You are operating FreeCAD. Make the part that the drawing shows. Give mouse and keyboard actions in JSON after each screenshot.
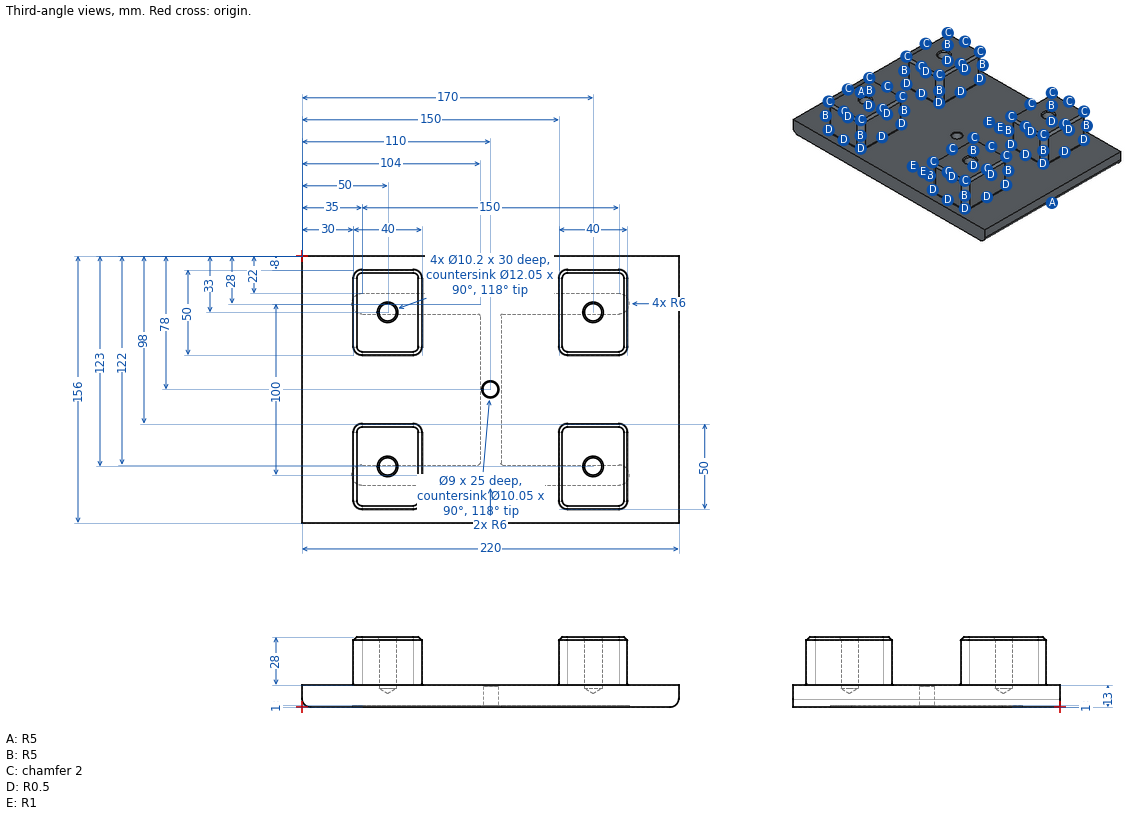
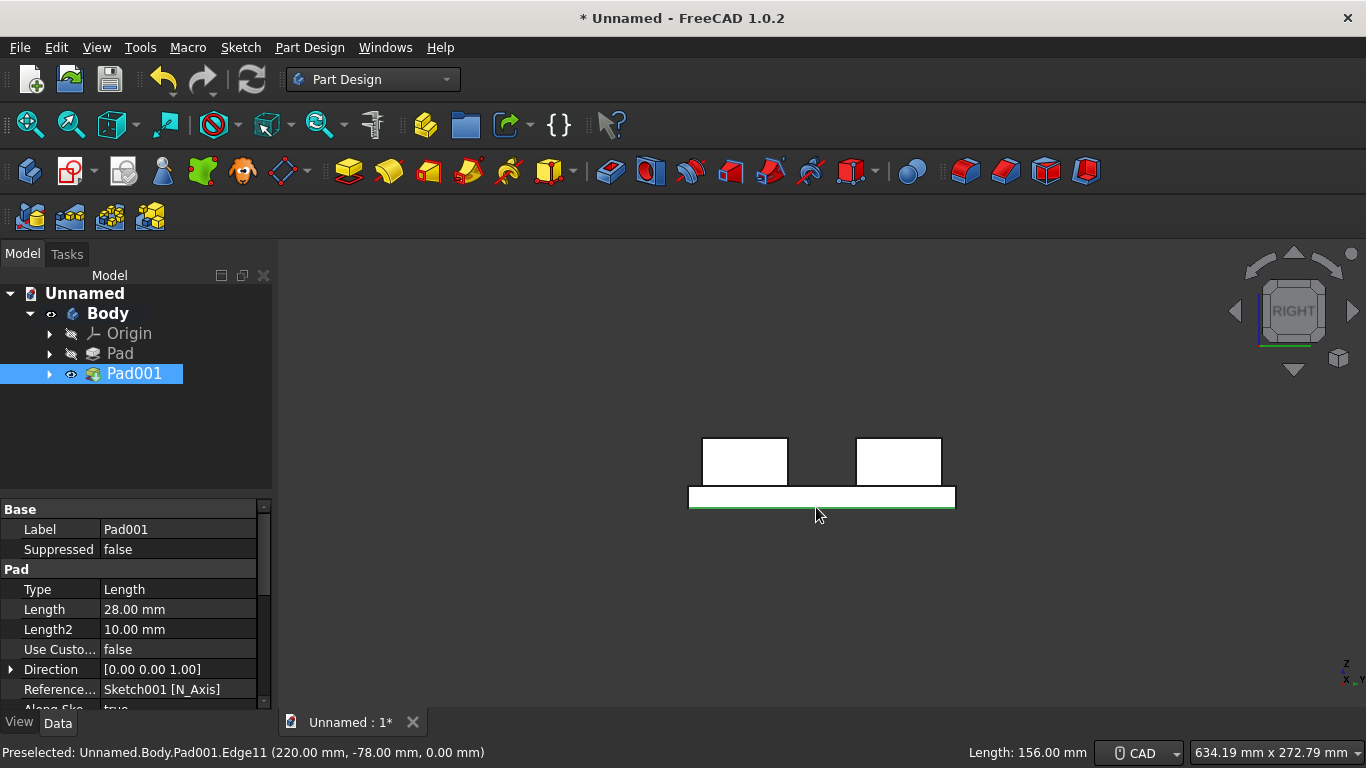
{"action": "key", "text": "5"}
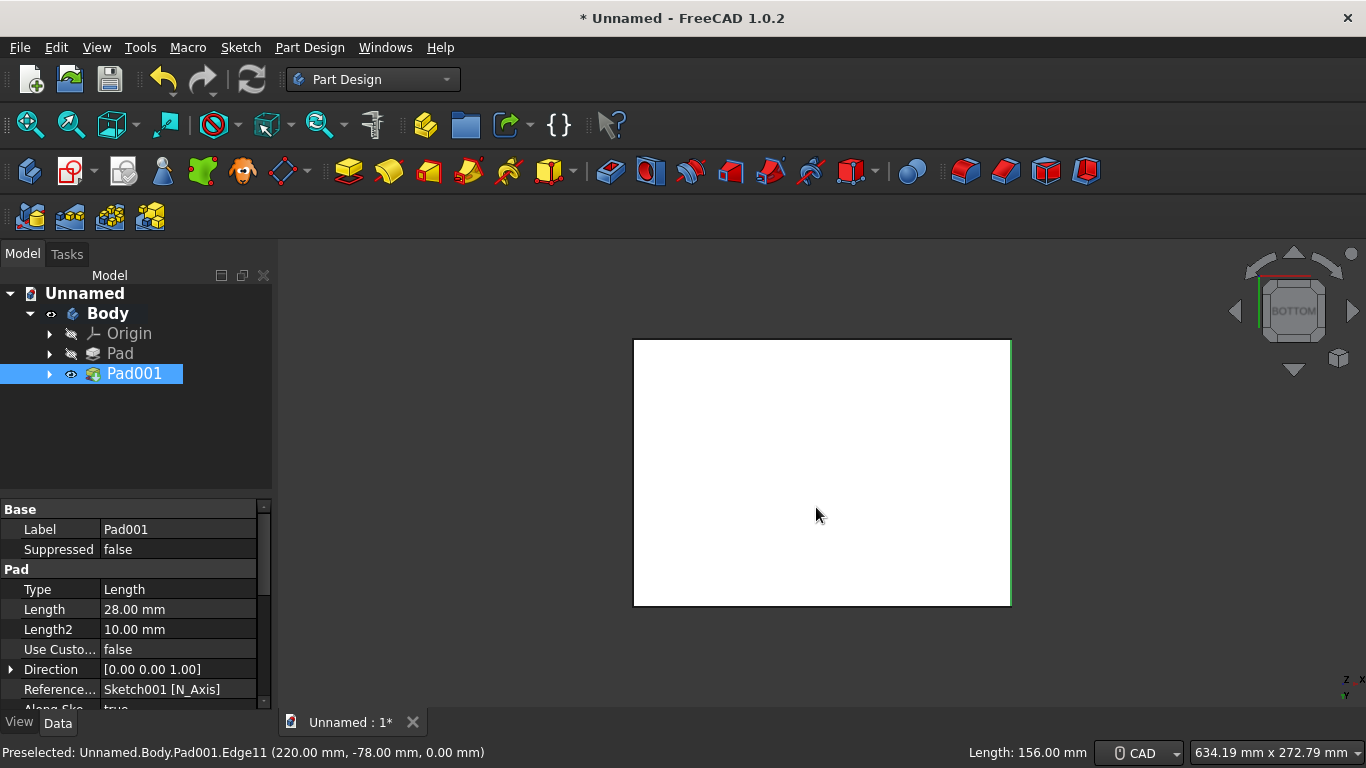
{"action": "left_click", "coordinate": [633, 472], "text": "ctrl"}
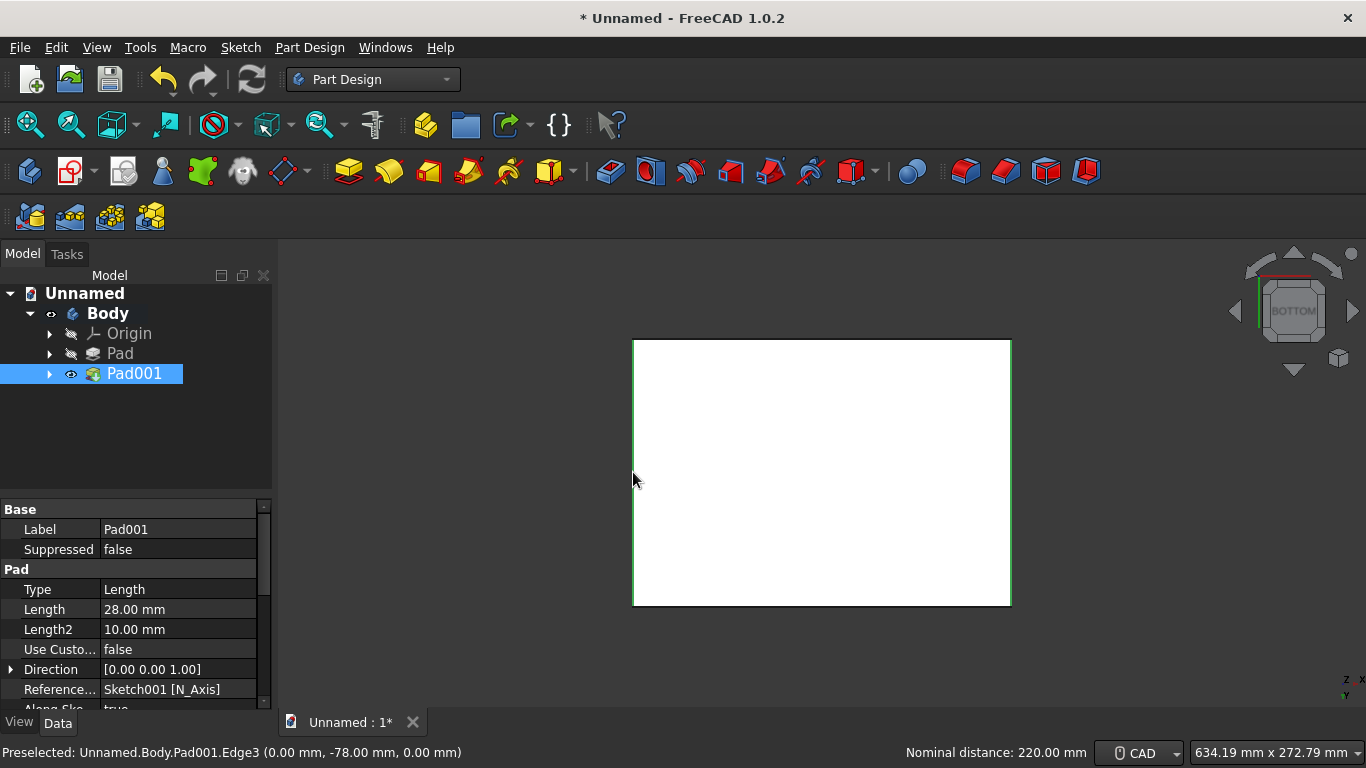
{"action": "left_click", "coordinate": [966, 172]}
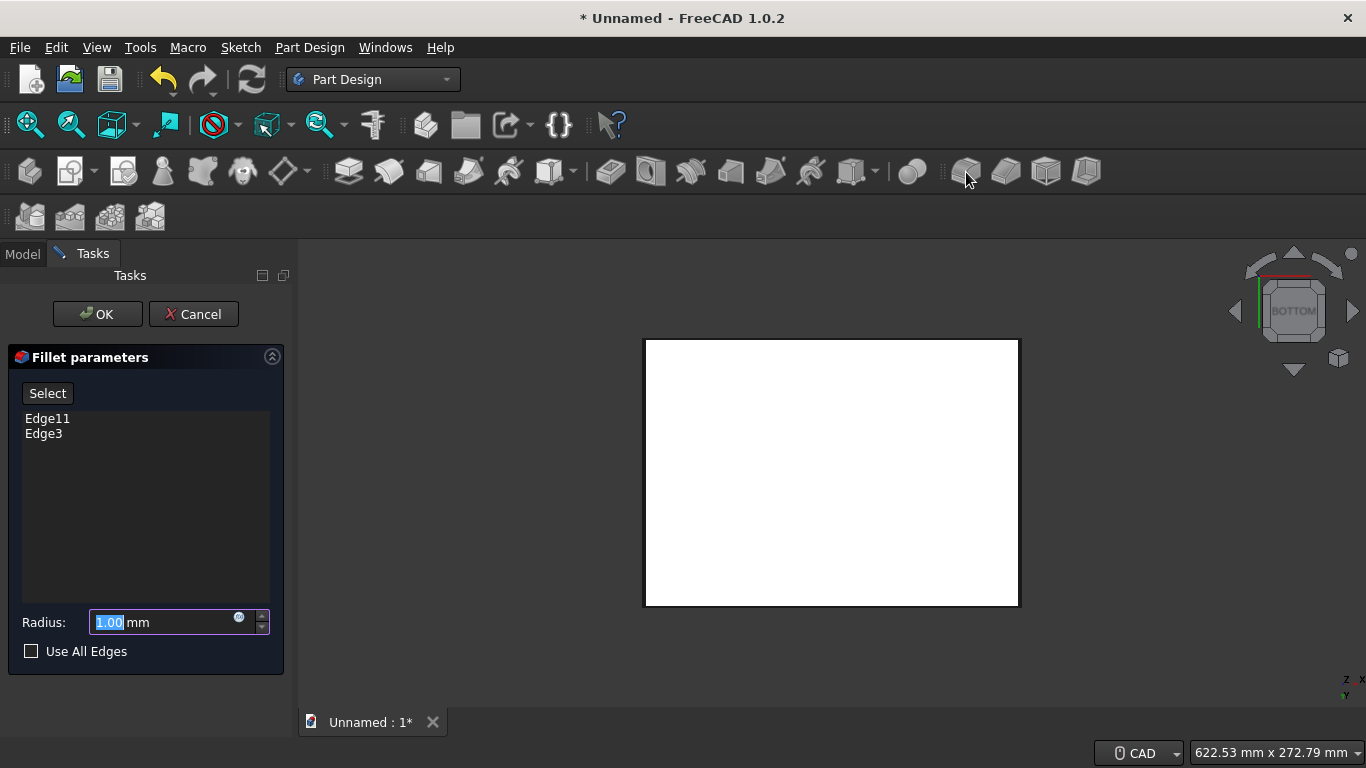
{"action": "type", "text": "5"}
{"action": "key", "text": "Tab"}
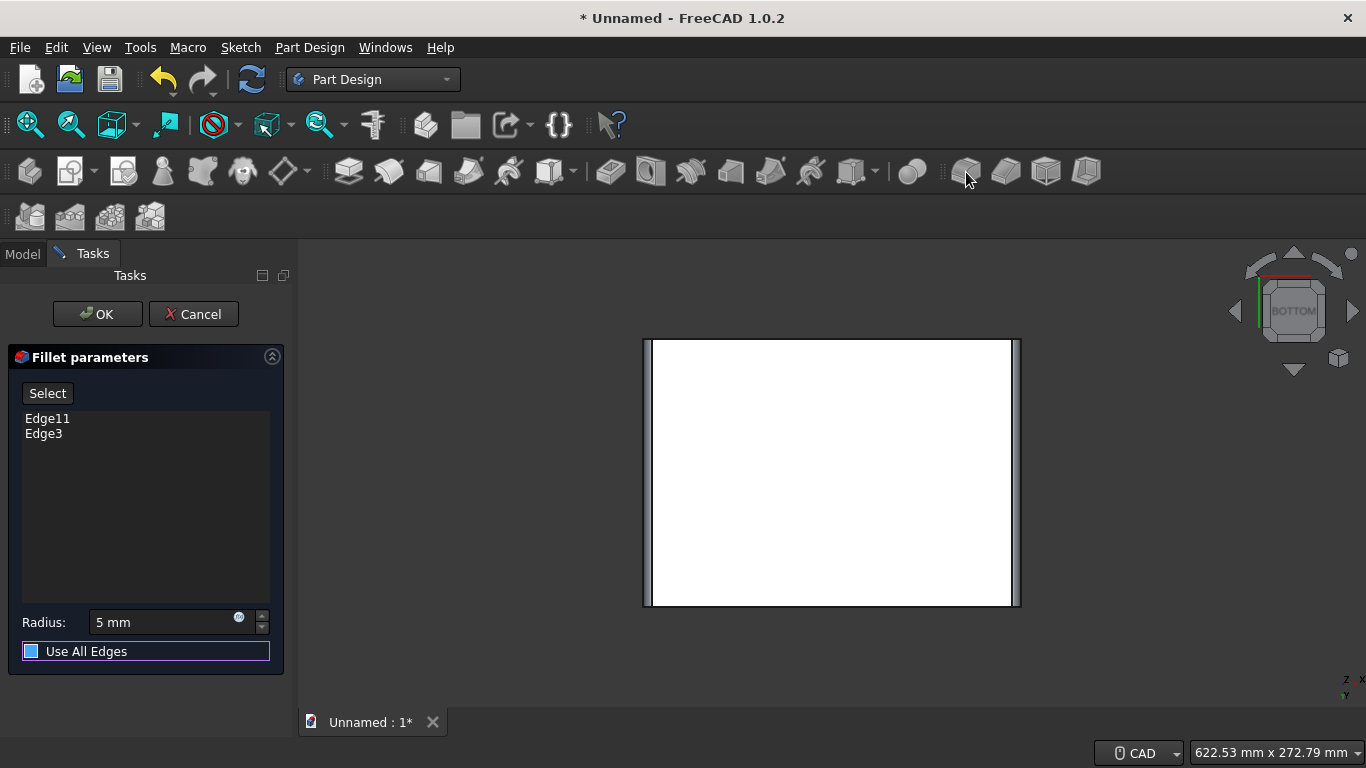
{"action": "left_click", "coordinate": [98, 314]}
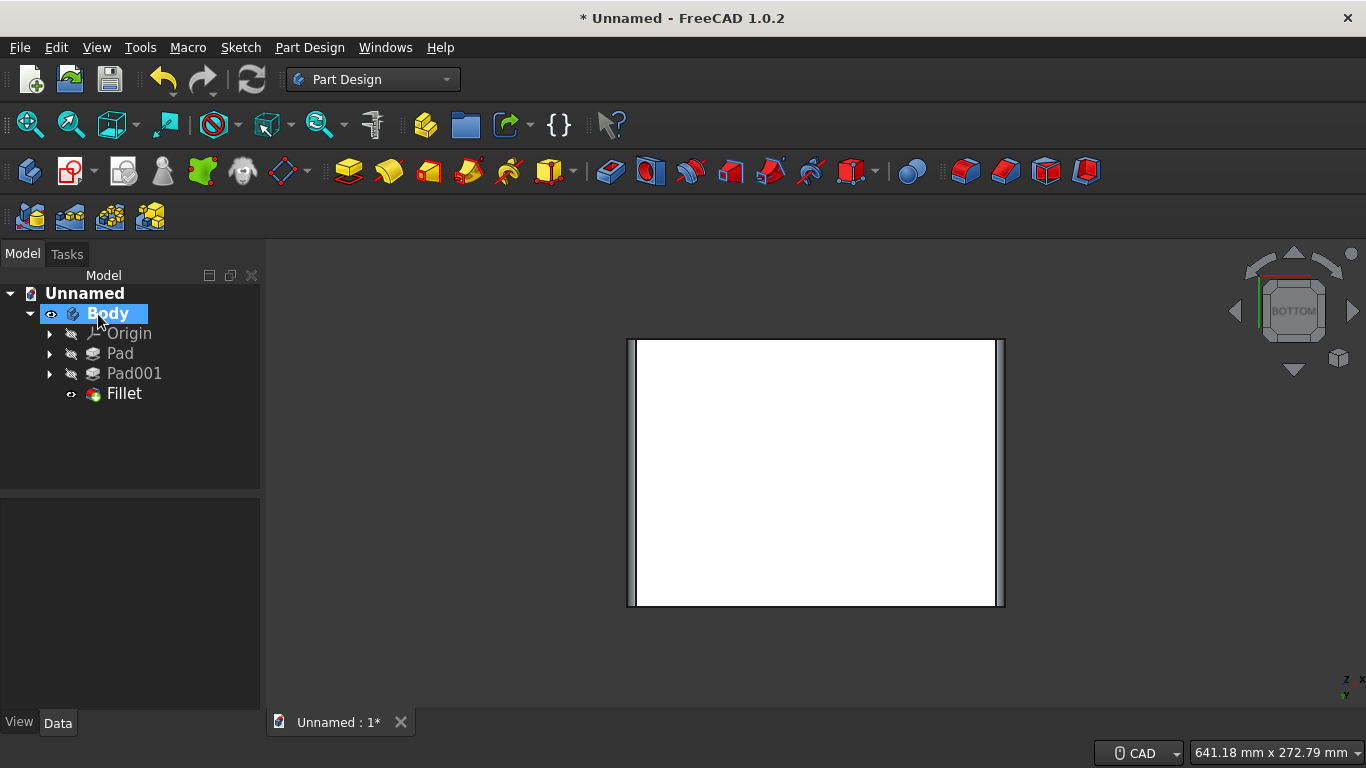
{"action": "key", "text": "0"}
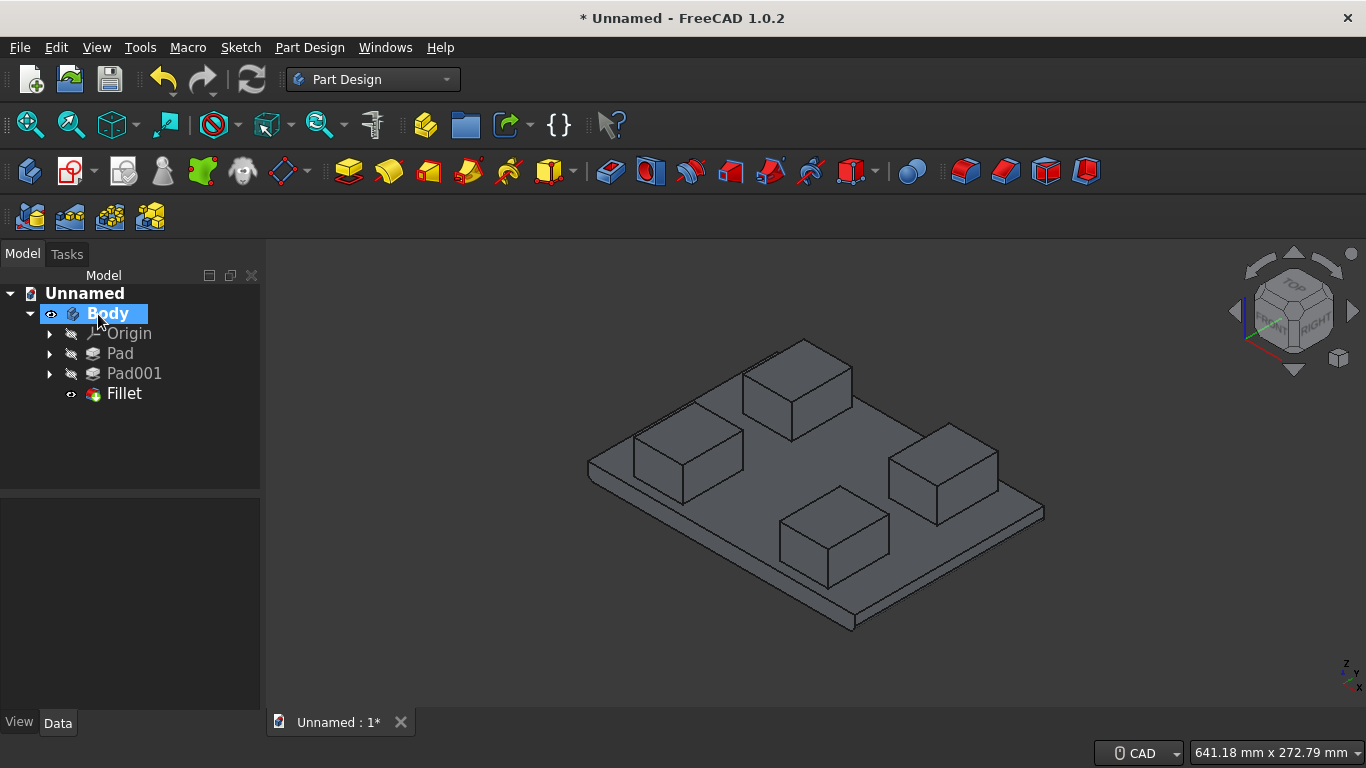
{"action": "left_click", "coordinate": [943, 454]}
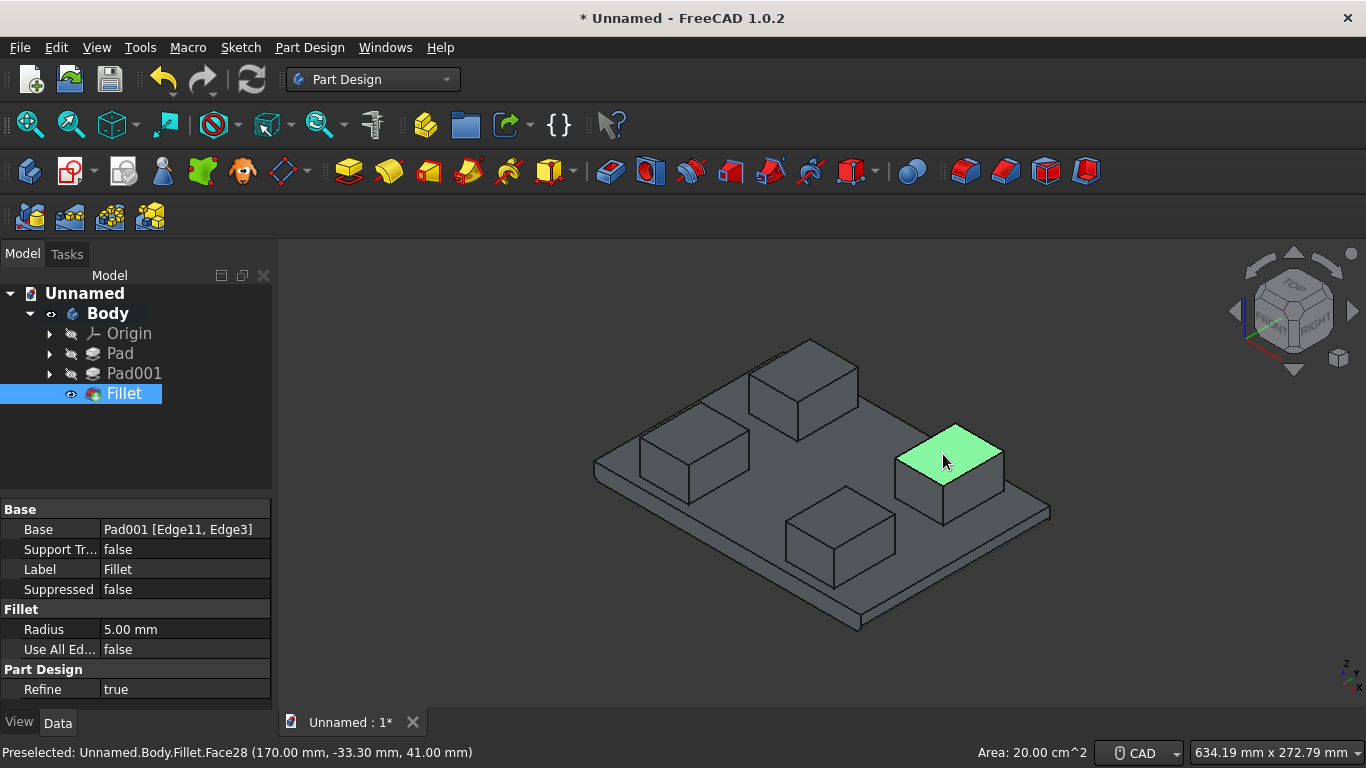
{"action": "left_click", "coordinate": [70, 172]}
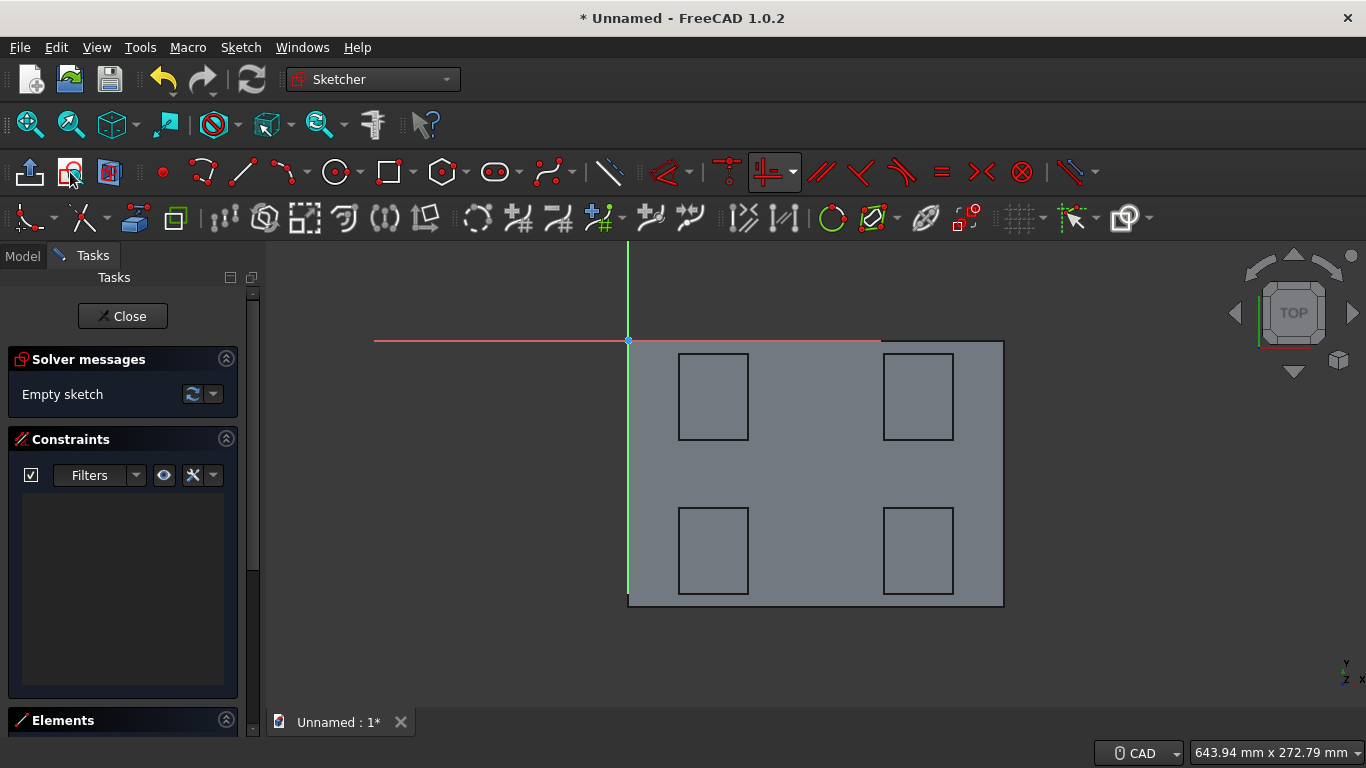
{"action": "left_click", "coordinate": [336, 172]}